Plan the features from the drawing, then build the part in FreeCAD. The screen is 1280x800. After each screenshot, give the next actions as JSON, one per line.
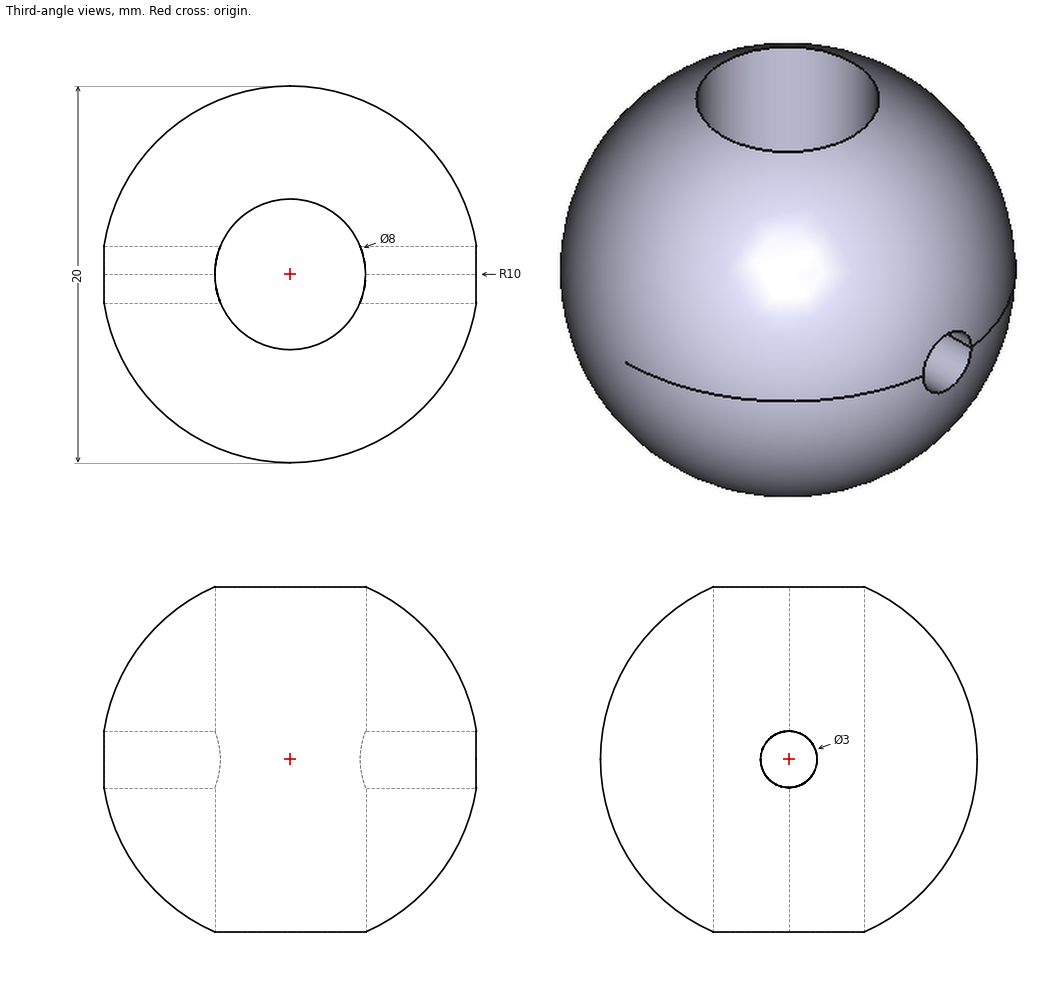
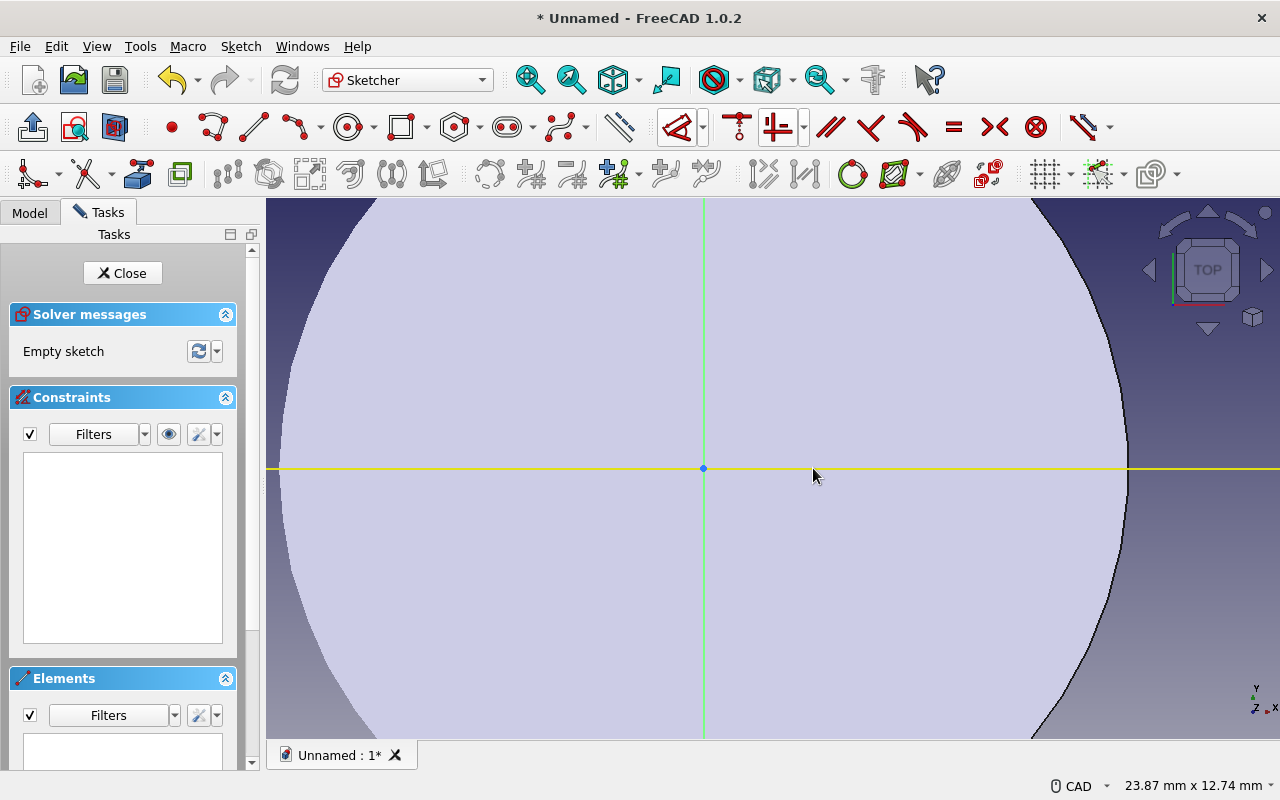
{"action": "left_click", "coordinate": [348, 128]}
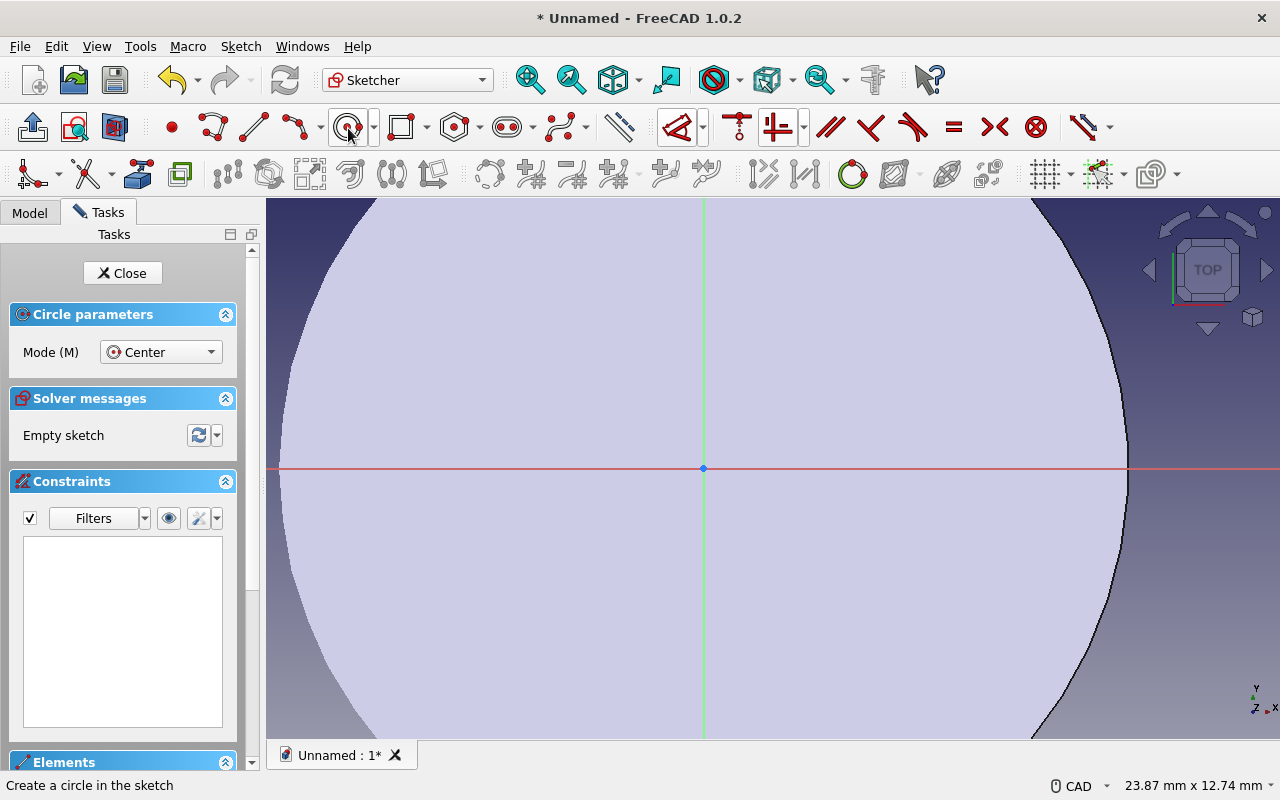
{"action": "left_click", "coordinate": [704, 468]}
{"action": "mouse_move", "coordinate": [824, 348]}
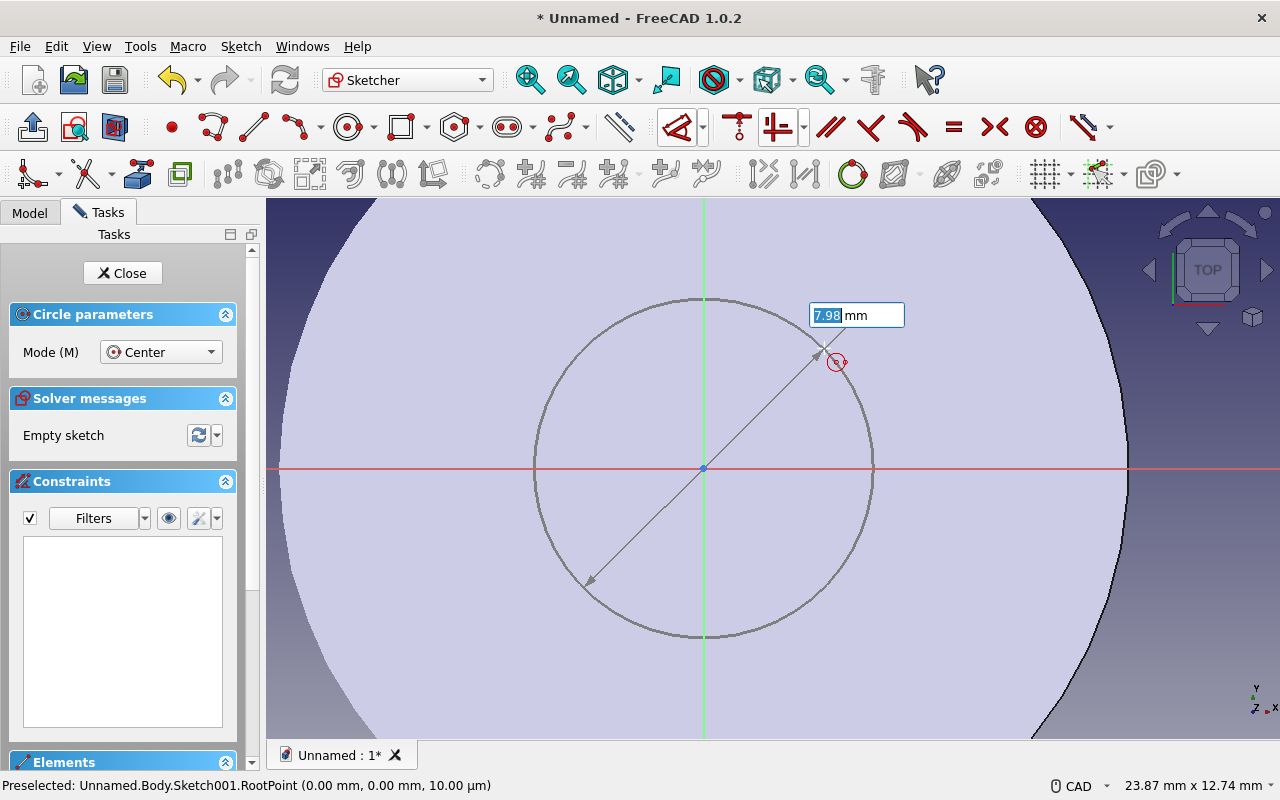
{"action": "type", "text": "8"}
{"action": "key", "text": "Return"}
{"action": "key", "text": "Escape"}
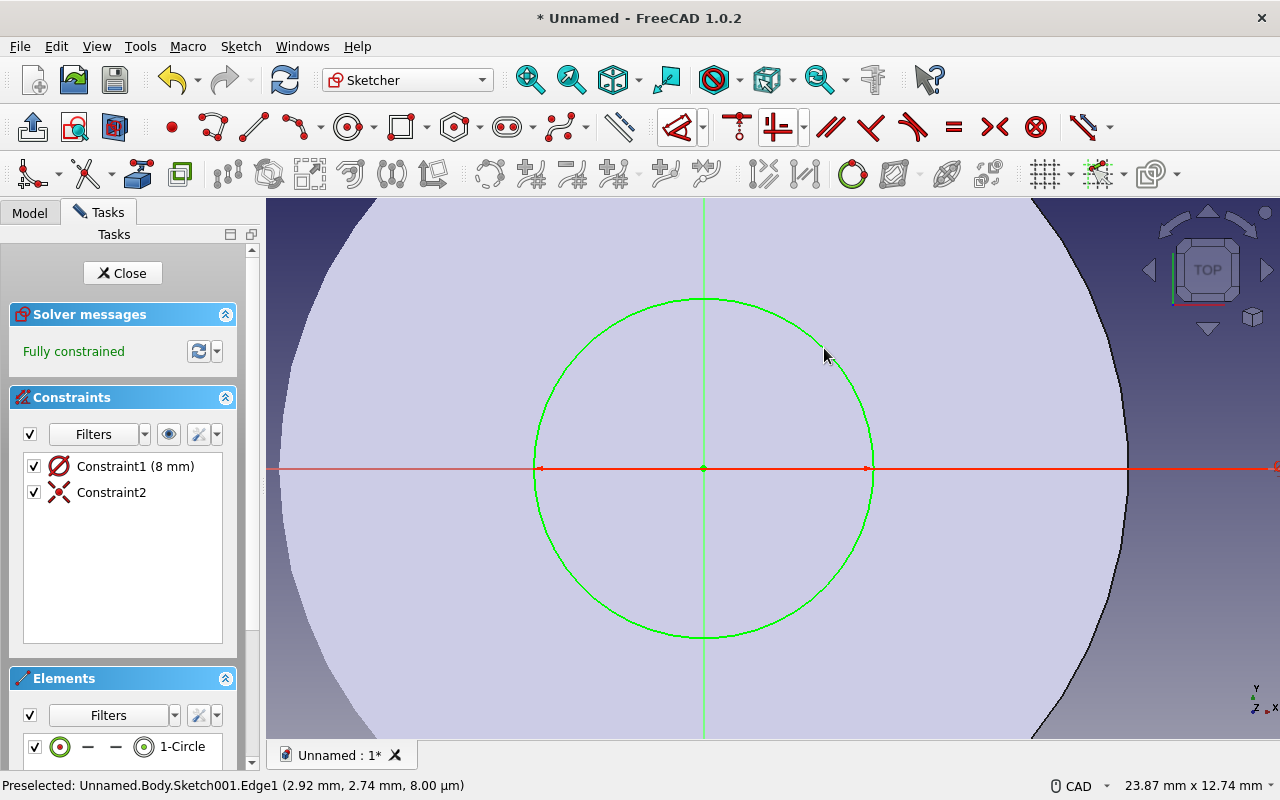
{"action": "left_click", "coordinate": [123, 273]}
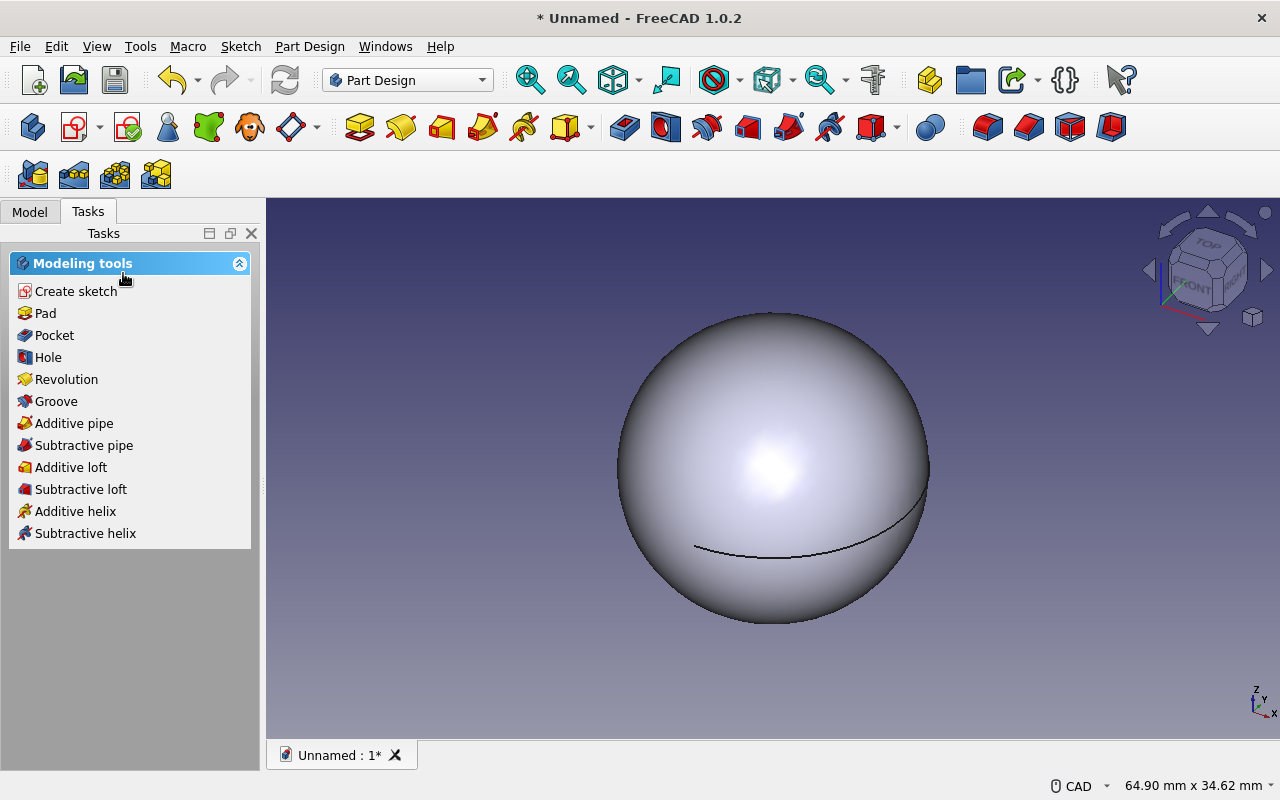
{"action": "left_click", "coordinate": [625, 128]}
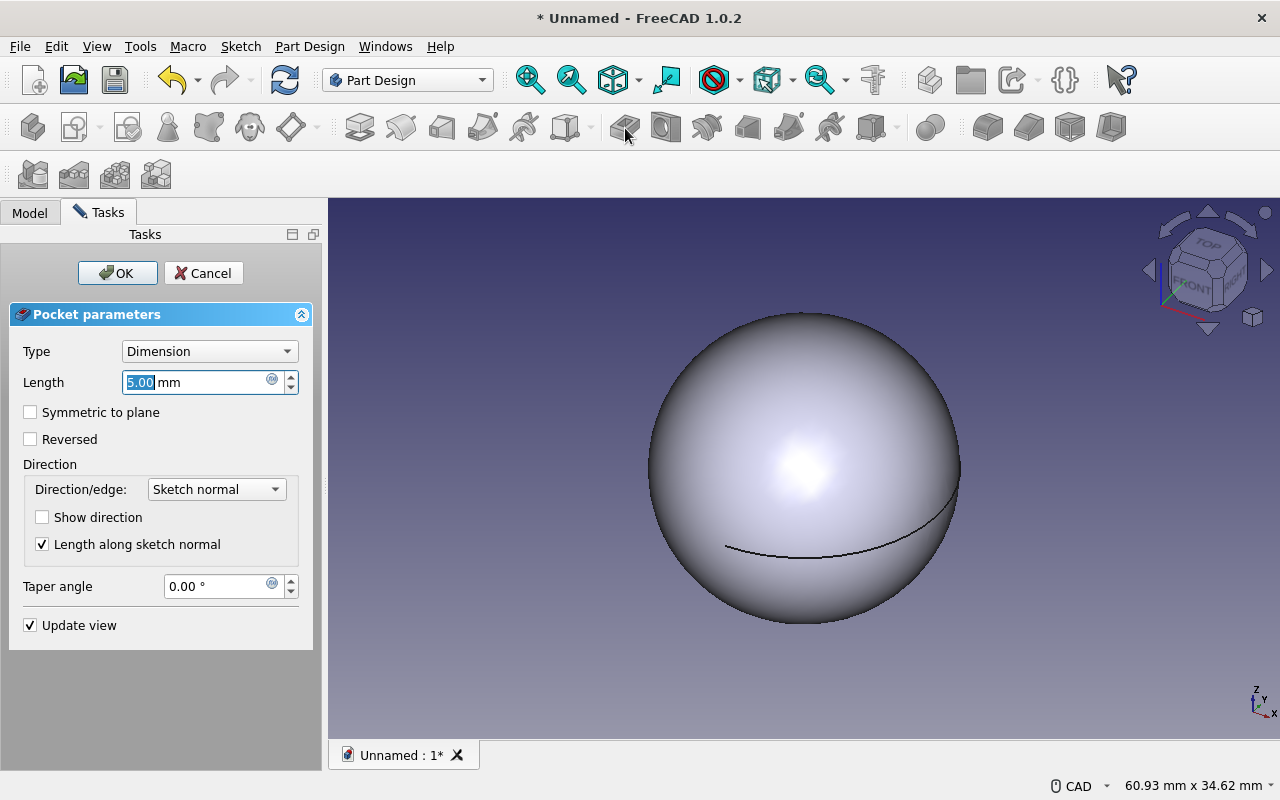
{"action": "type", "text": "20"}
{"action": "key", "text": "Tab"}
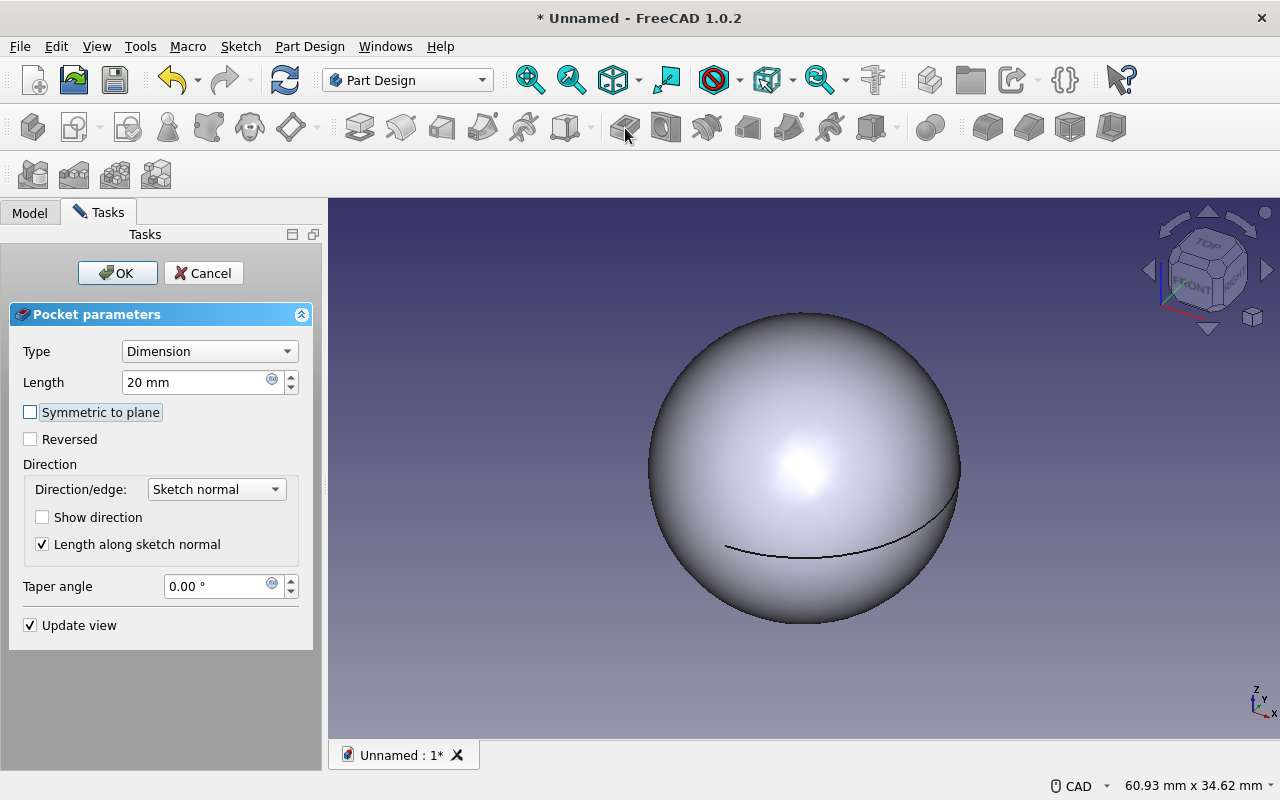
{"action": "left_click", "coordinate": [31, 412]}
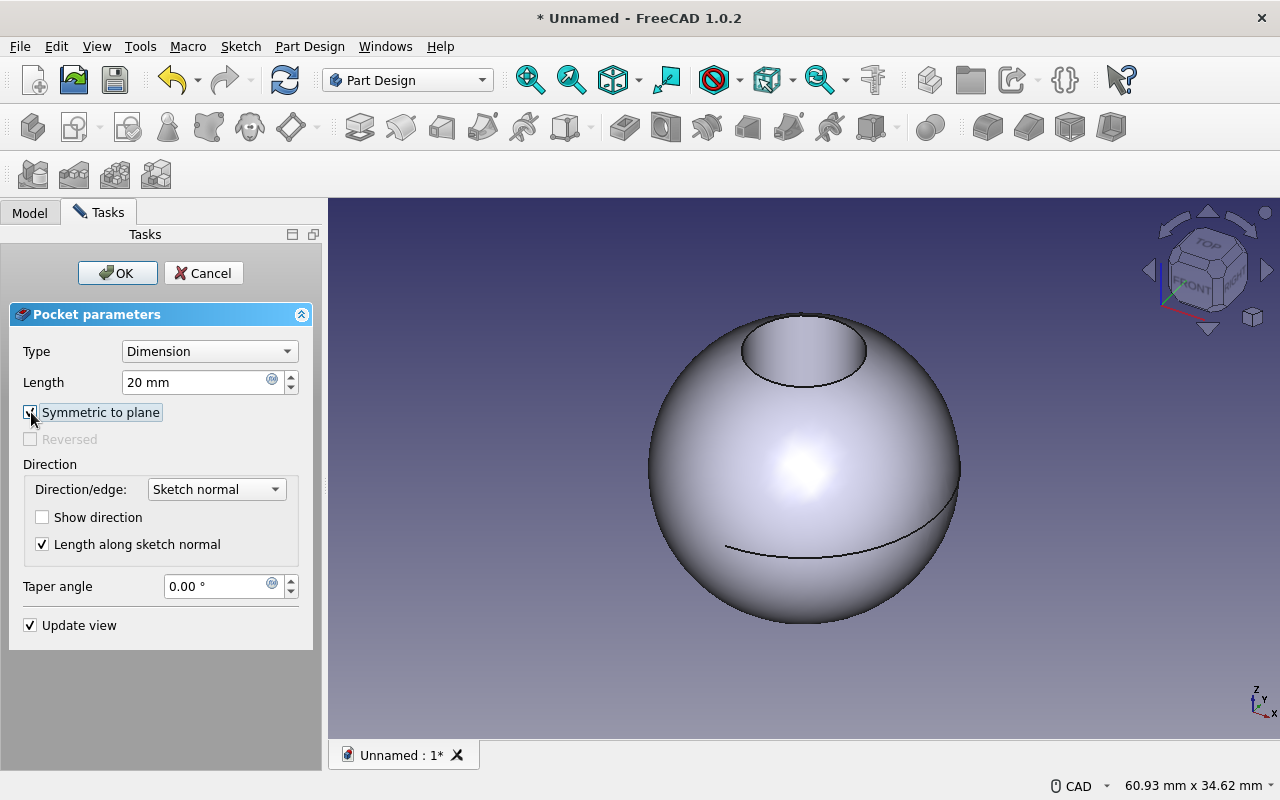
{"action": "left_click", "coordinate": [118, 273]}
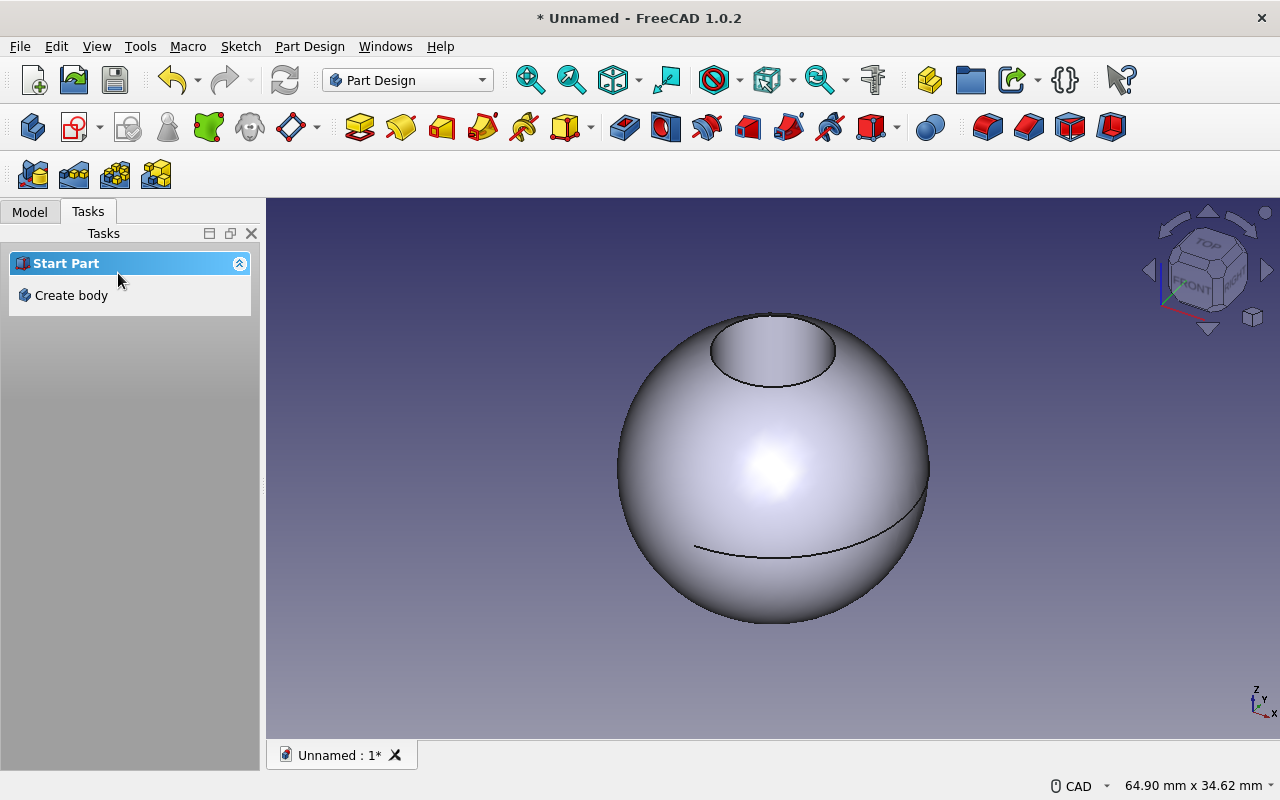
{"action": "left_click", "coordinate": [74, 128]}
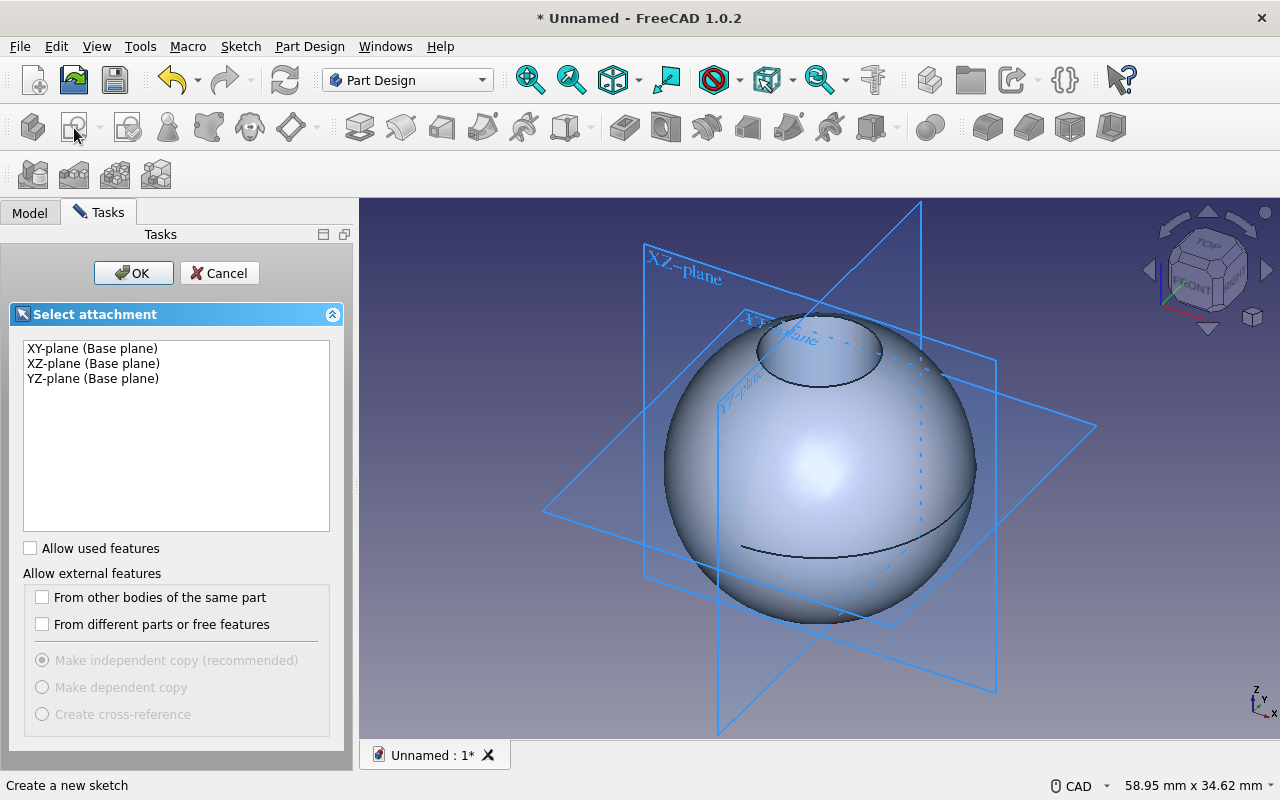
{"action": "left_click", "coordinate": [84, 378]}